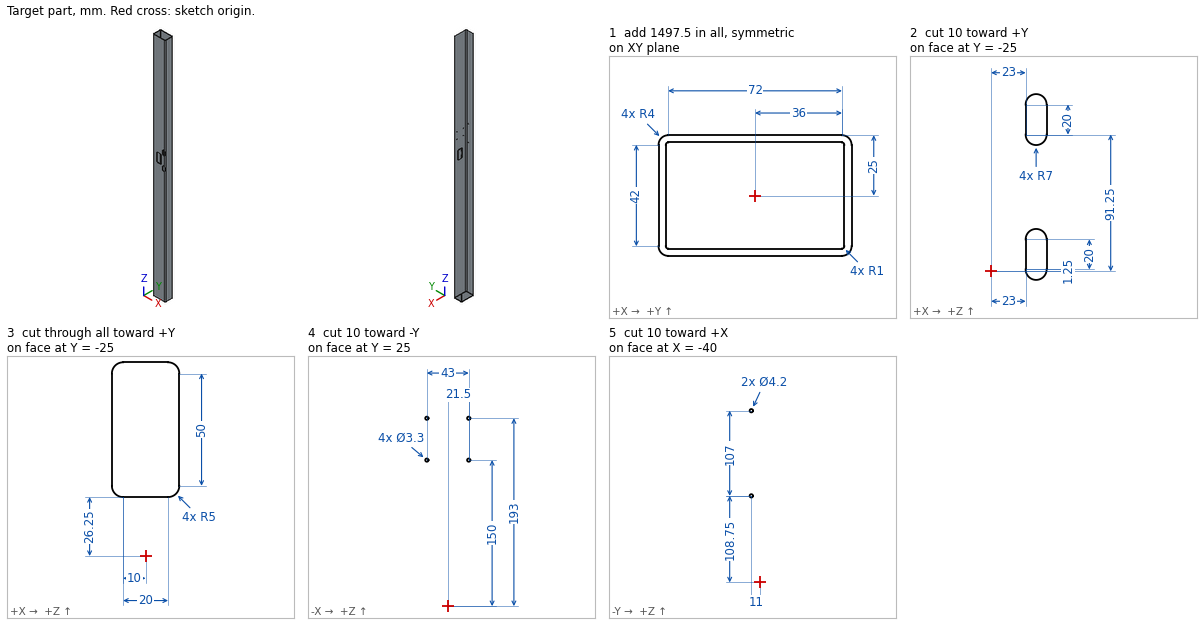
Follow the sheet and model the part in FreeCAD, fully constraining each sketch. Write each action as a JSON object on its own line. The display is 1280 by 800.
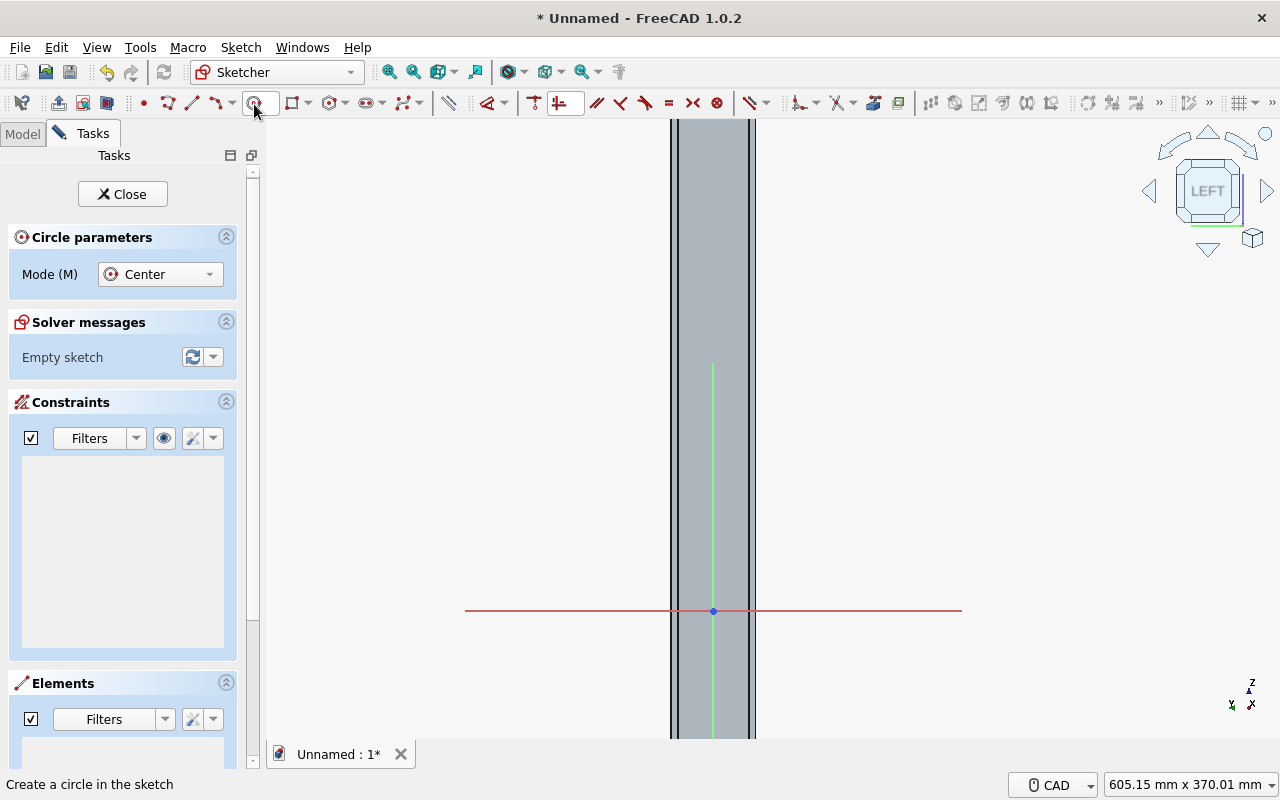
{"action": "scroll", "coordinate": [695, 429], "scroll_direction": "up", "scroll_amount": 10}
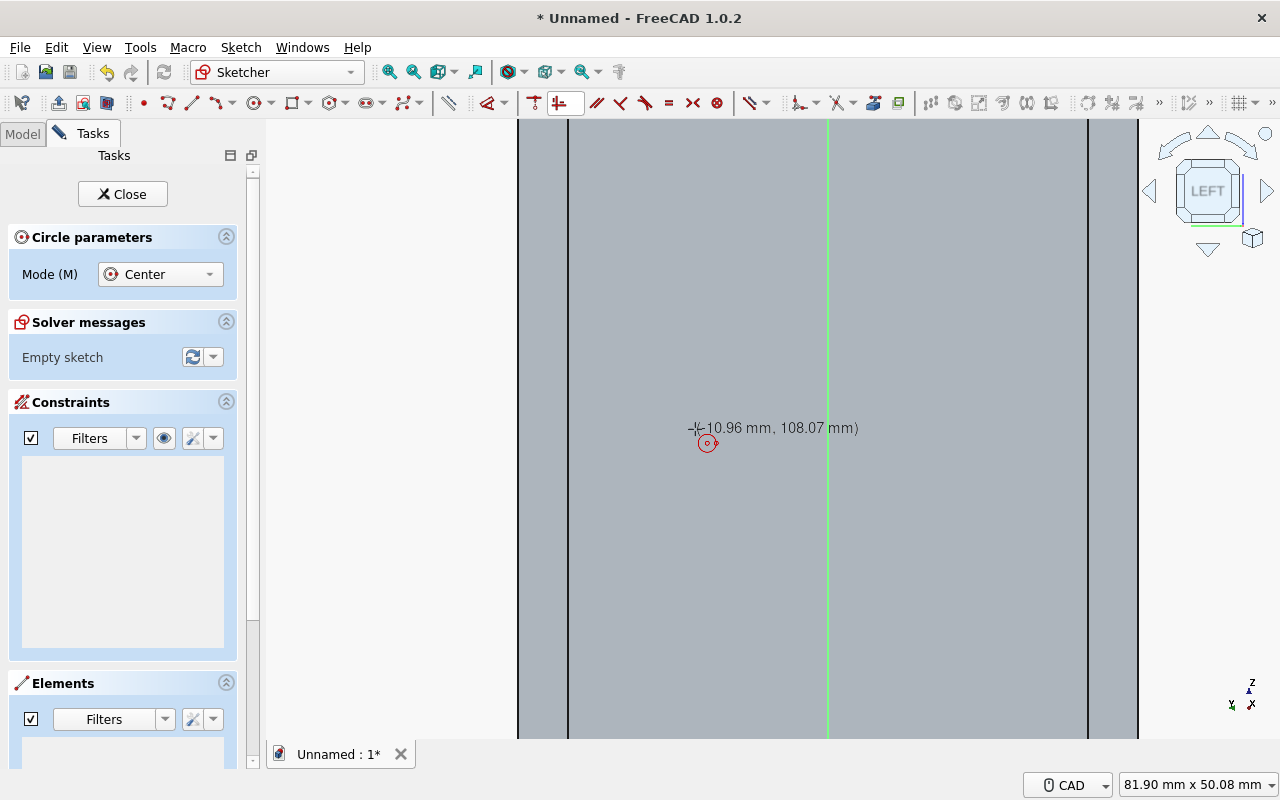
{"action": "scroll", "coordinate": [698, 430], "scroll_direction": "down", "scroll_amount": 10}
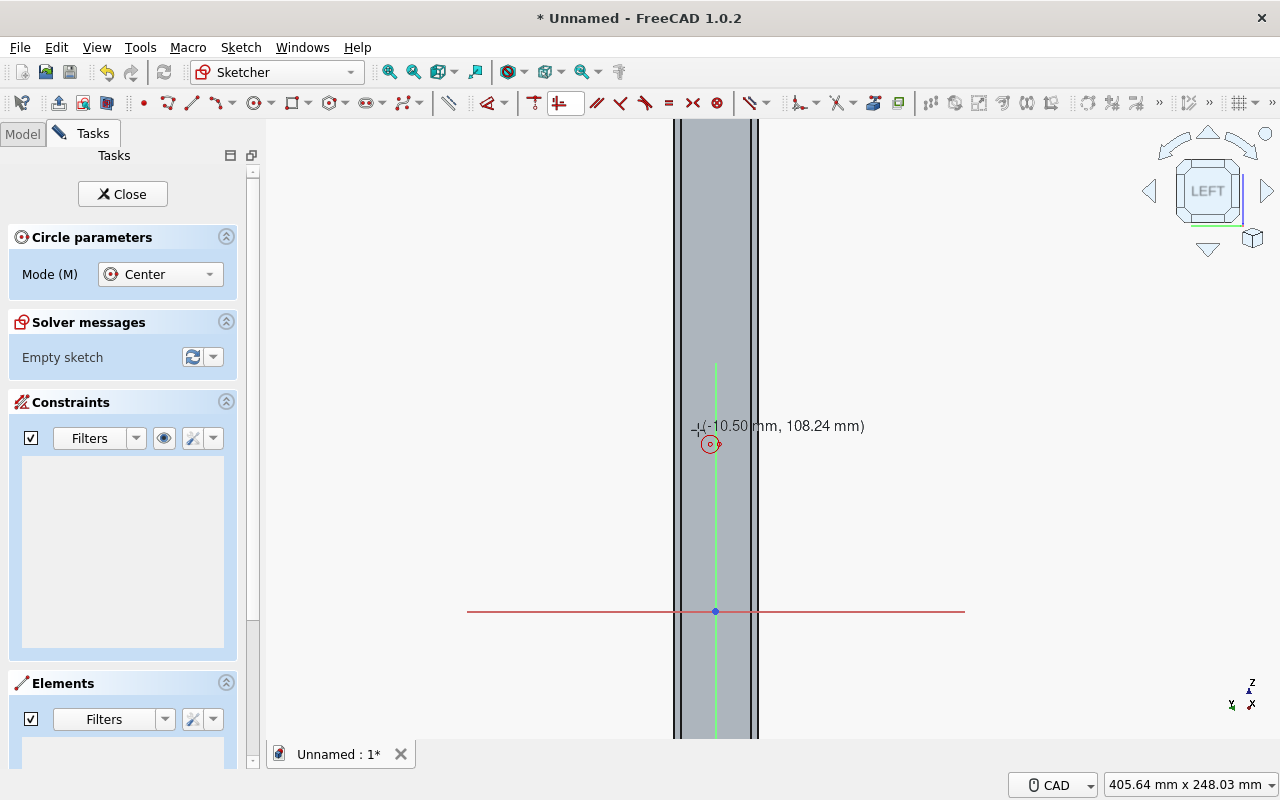
{"action": "left_click", "coordinate": [698, 430]}
{"action": "mouse_move", "coordinate": [700, 427]}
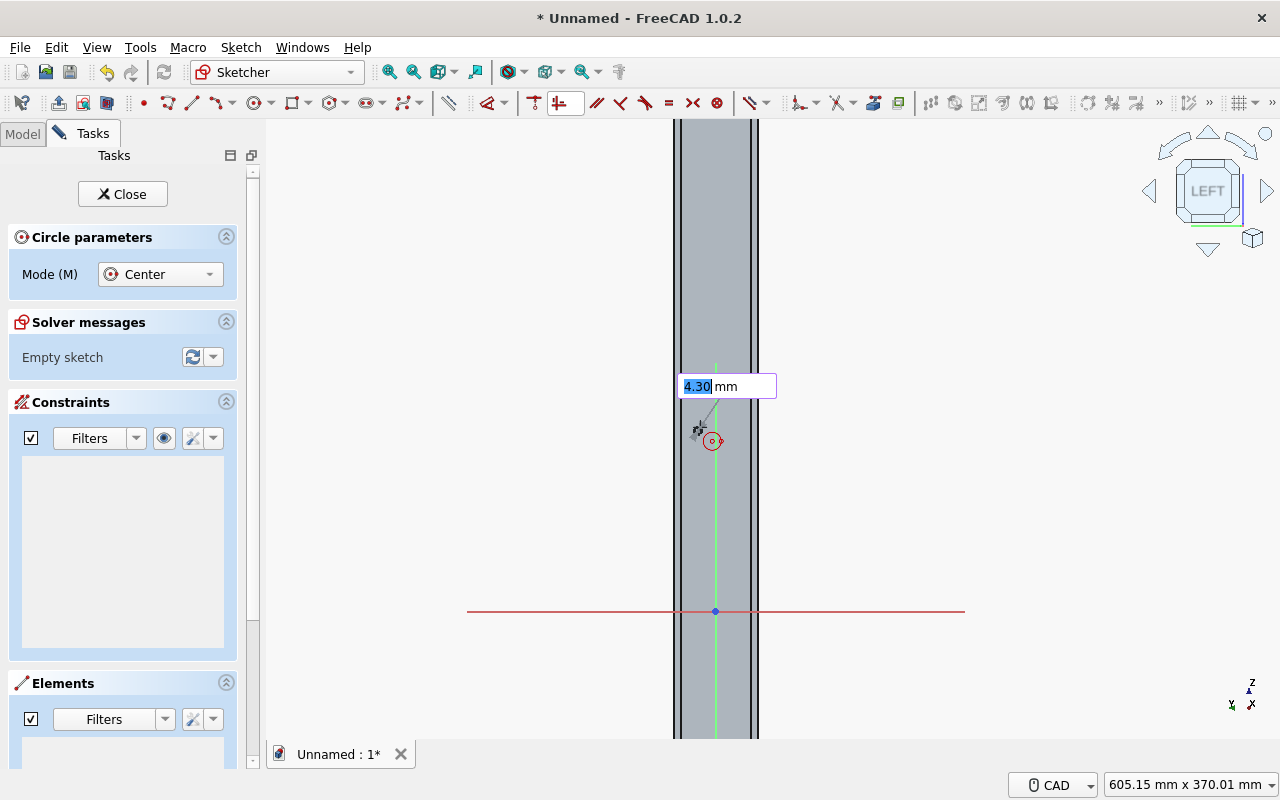
{"action": "type", "text": "4.2"}
{"action": "key", "text": "Return"}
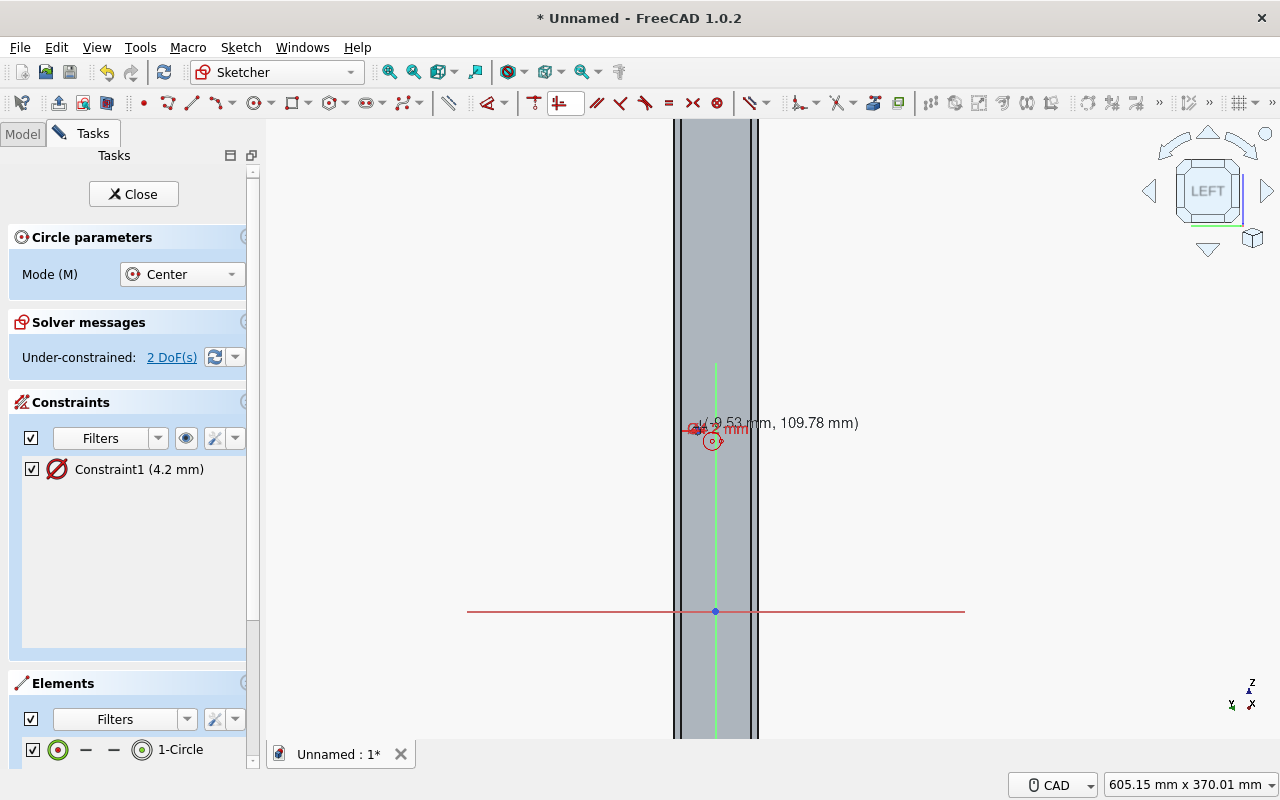
{"action": "scroll", "coordinate": [698, 250], "scroll_direction": "up", "scroll_amount": 10}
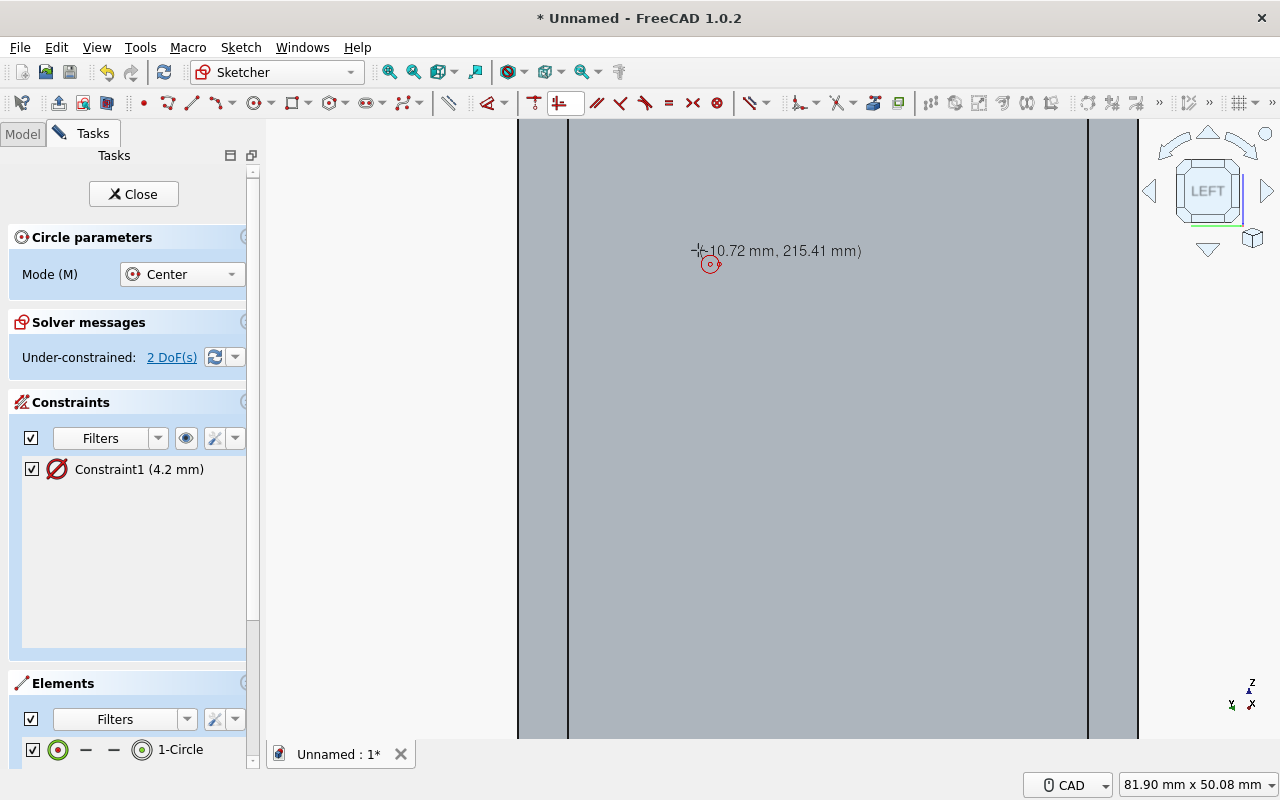
{"action": "scroll", "coordinate": [698, 250], "scroll_direction": "down", "scroll_amount": 10}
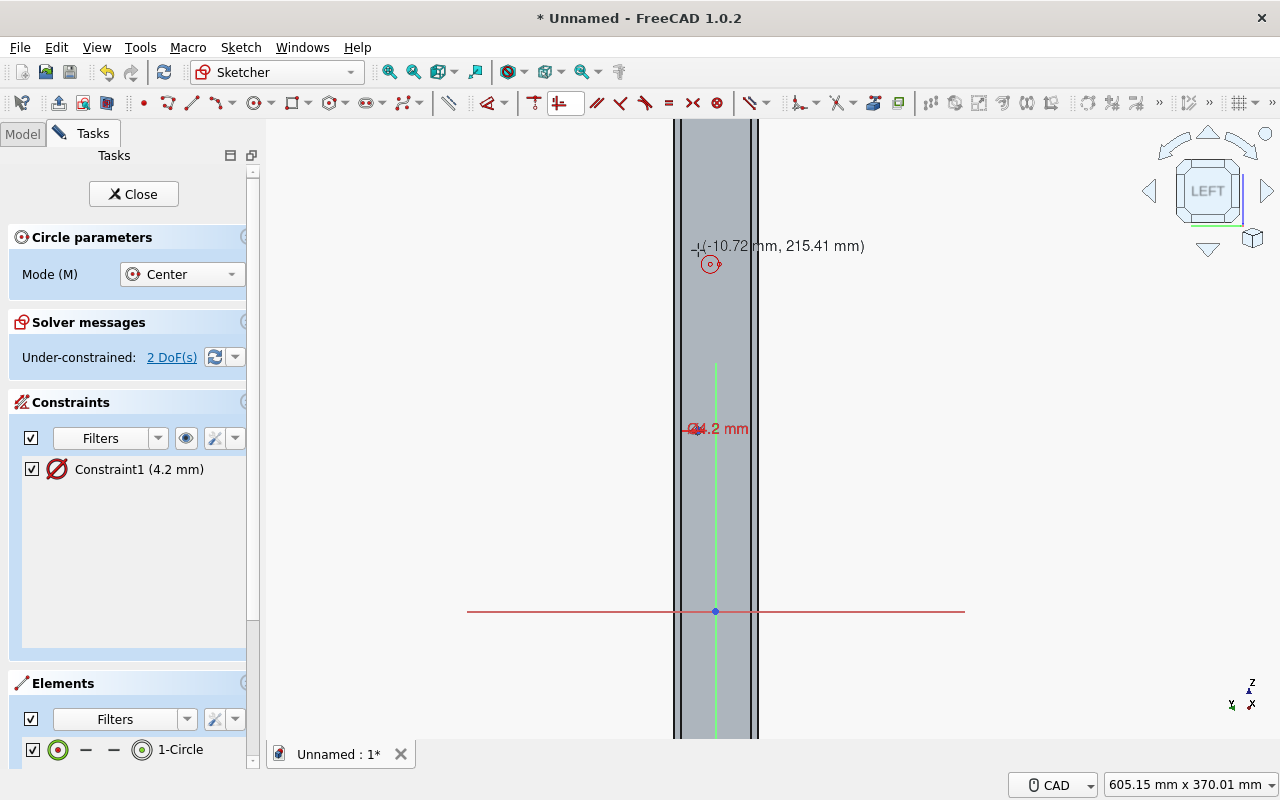
{"action": "left_click", "coordinate": [698, 250]}
{"action": "mouse_move", "coordinate": [700, 248]}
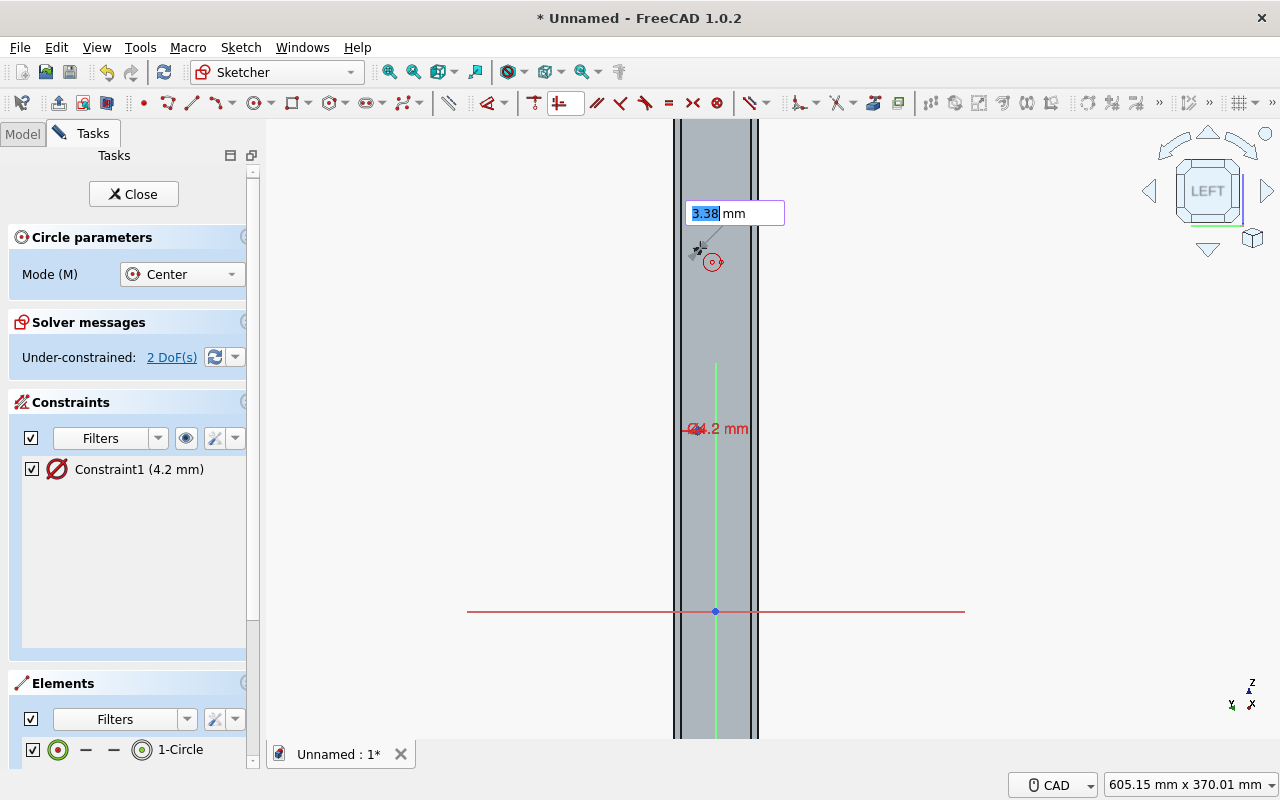
{"action": "type", "text": "4.2"}
{"action": "key", "text": "Return"}
{"action": "key", "text": "Escape"}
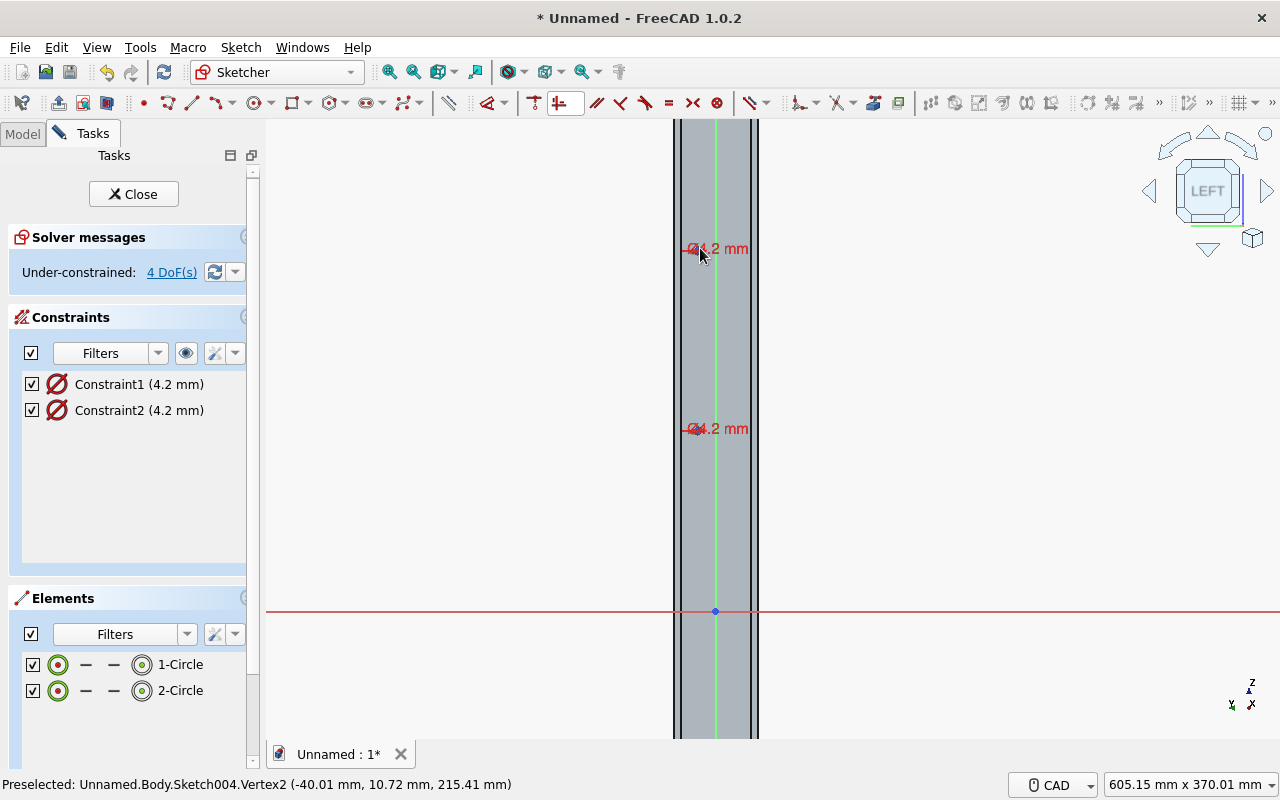
{"action": "left_click", "coordinate": [698, 431]}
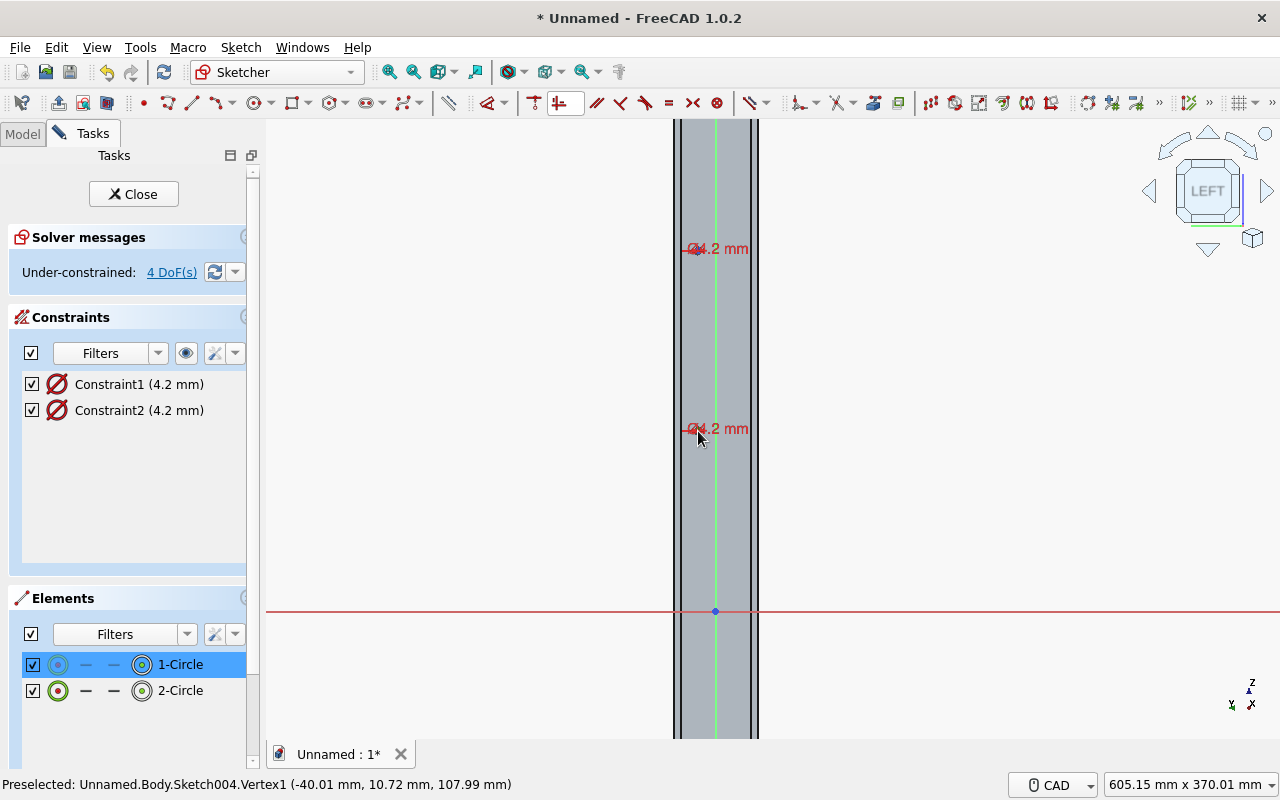
{"action": "left_click", "coordinate": [698, 251]}